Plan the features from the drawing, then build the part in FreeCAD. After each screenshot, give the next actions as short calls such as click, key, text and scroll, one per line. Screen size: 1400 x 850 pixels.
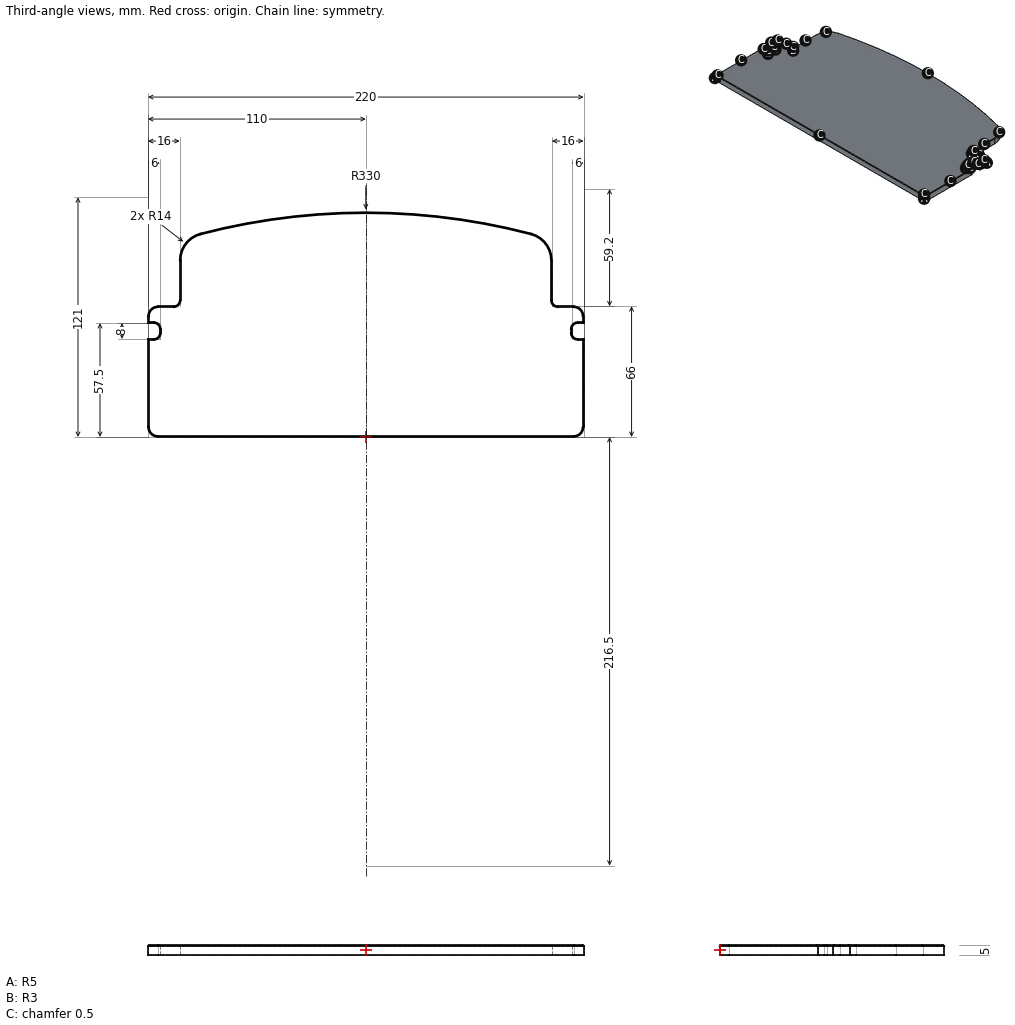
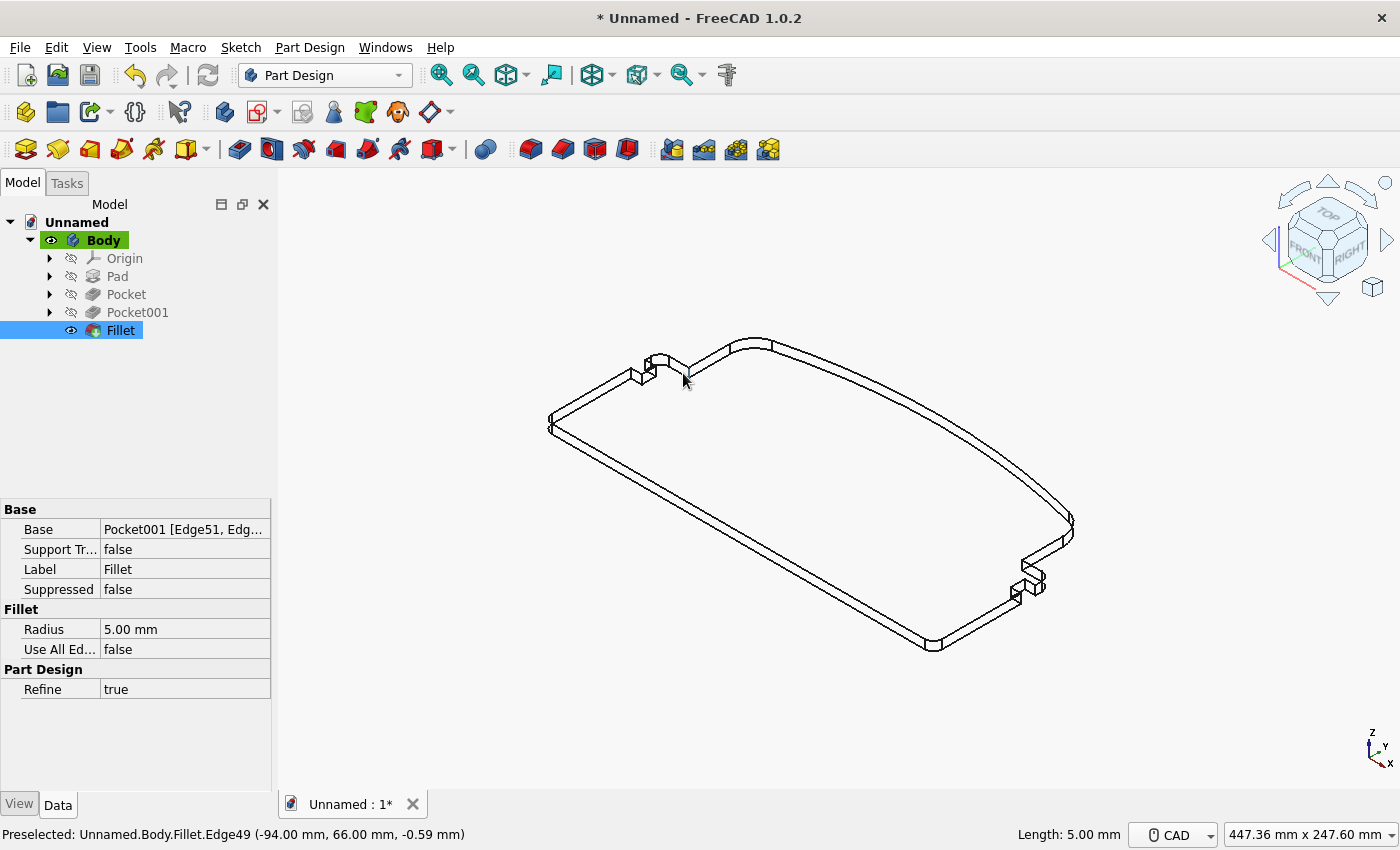
click(1022, 567, ctrl)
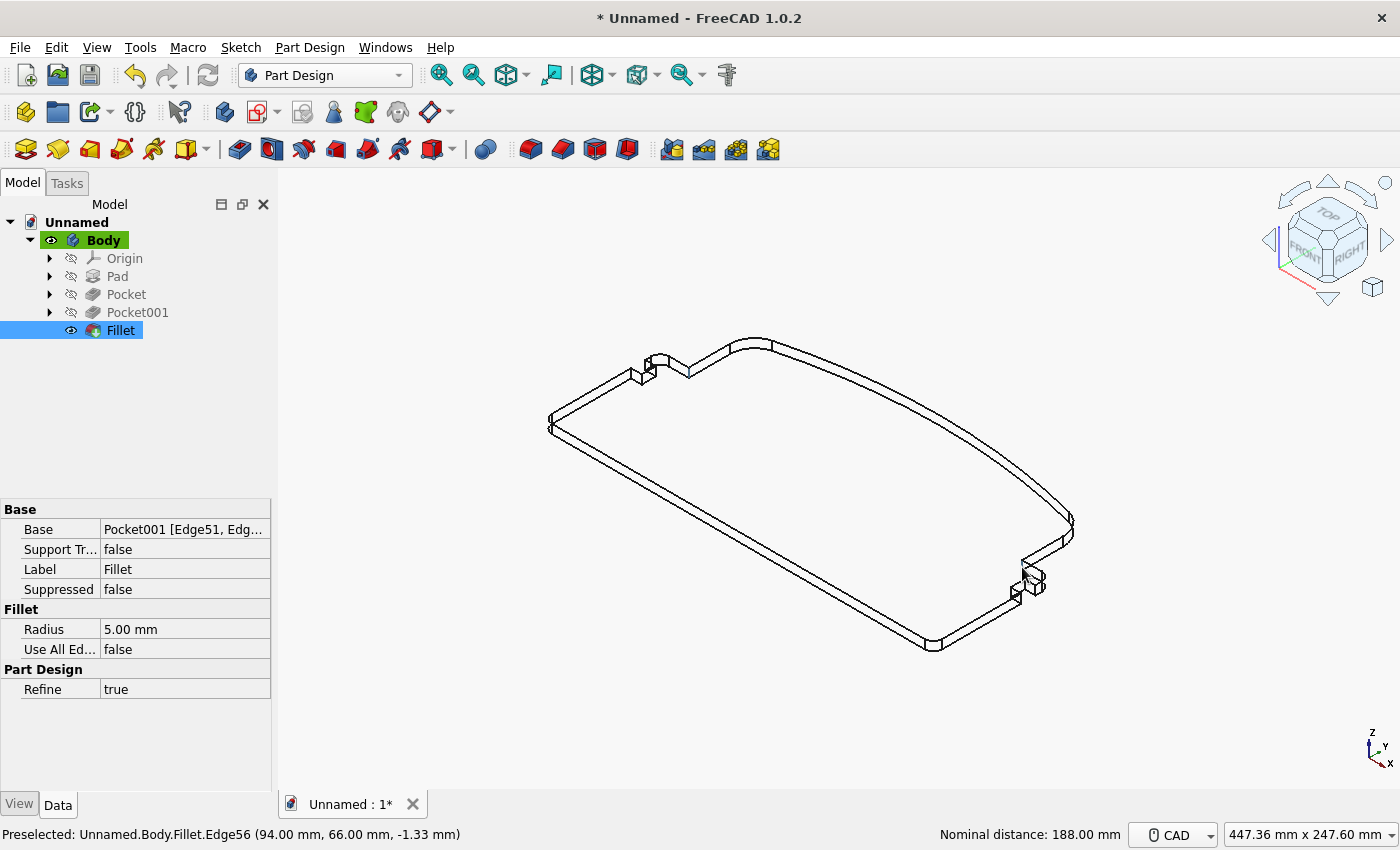
click(656, 373, ctrl)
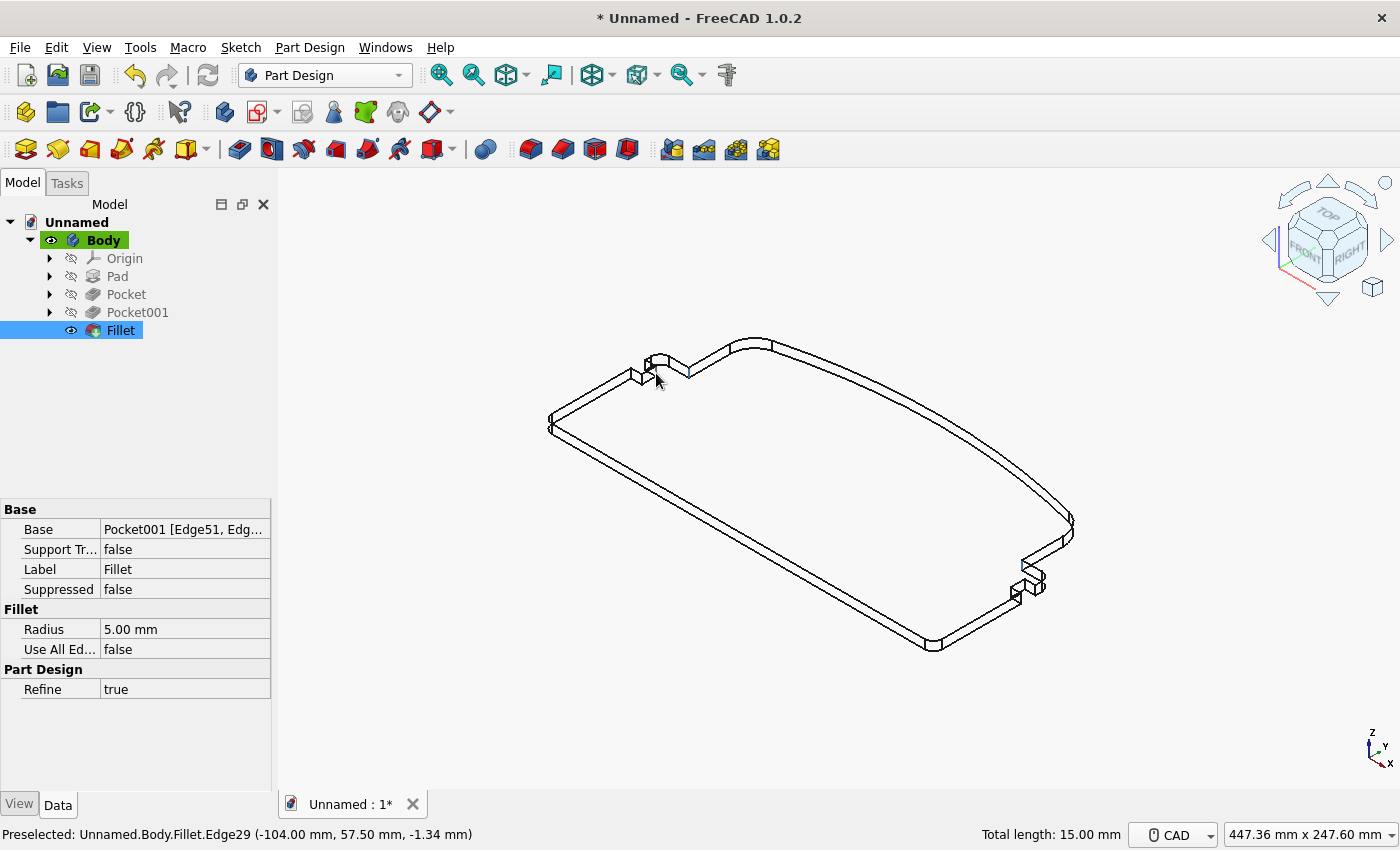
click(642, 380, ctrl)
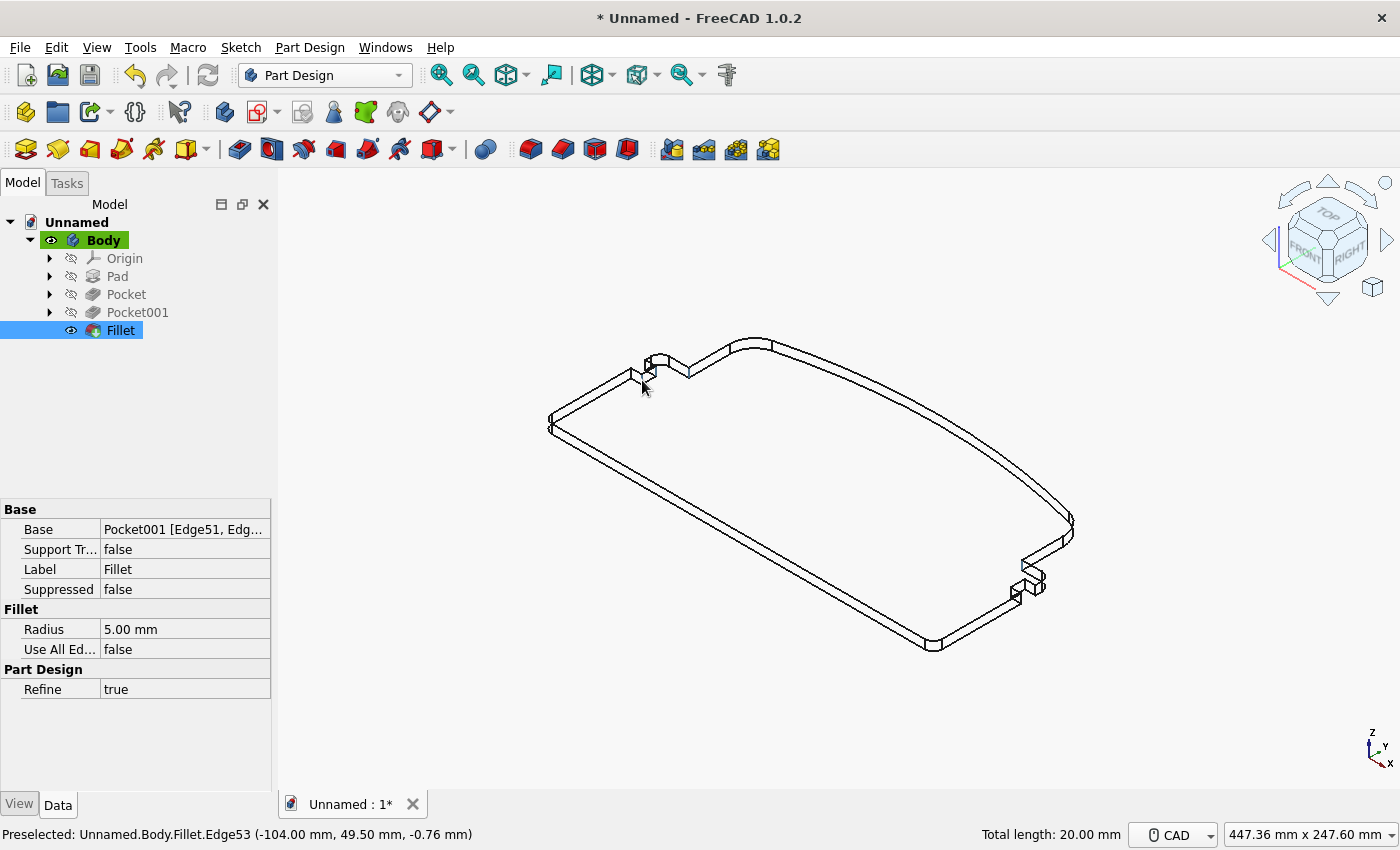
click(1025, 586, ctrl)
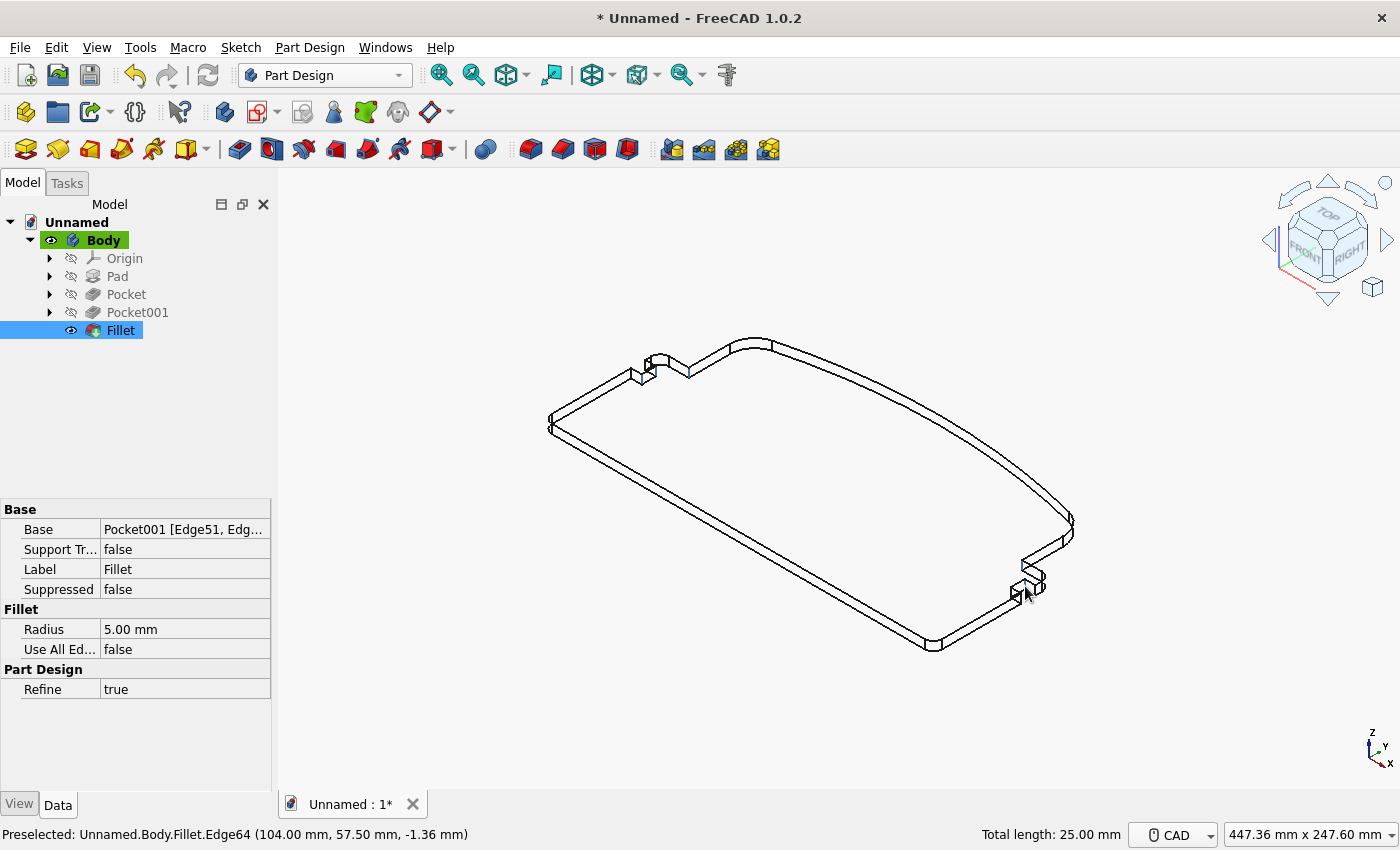
scroll(1011, 591, up, 6)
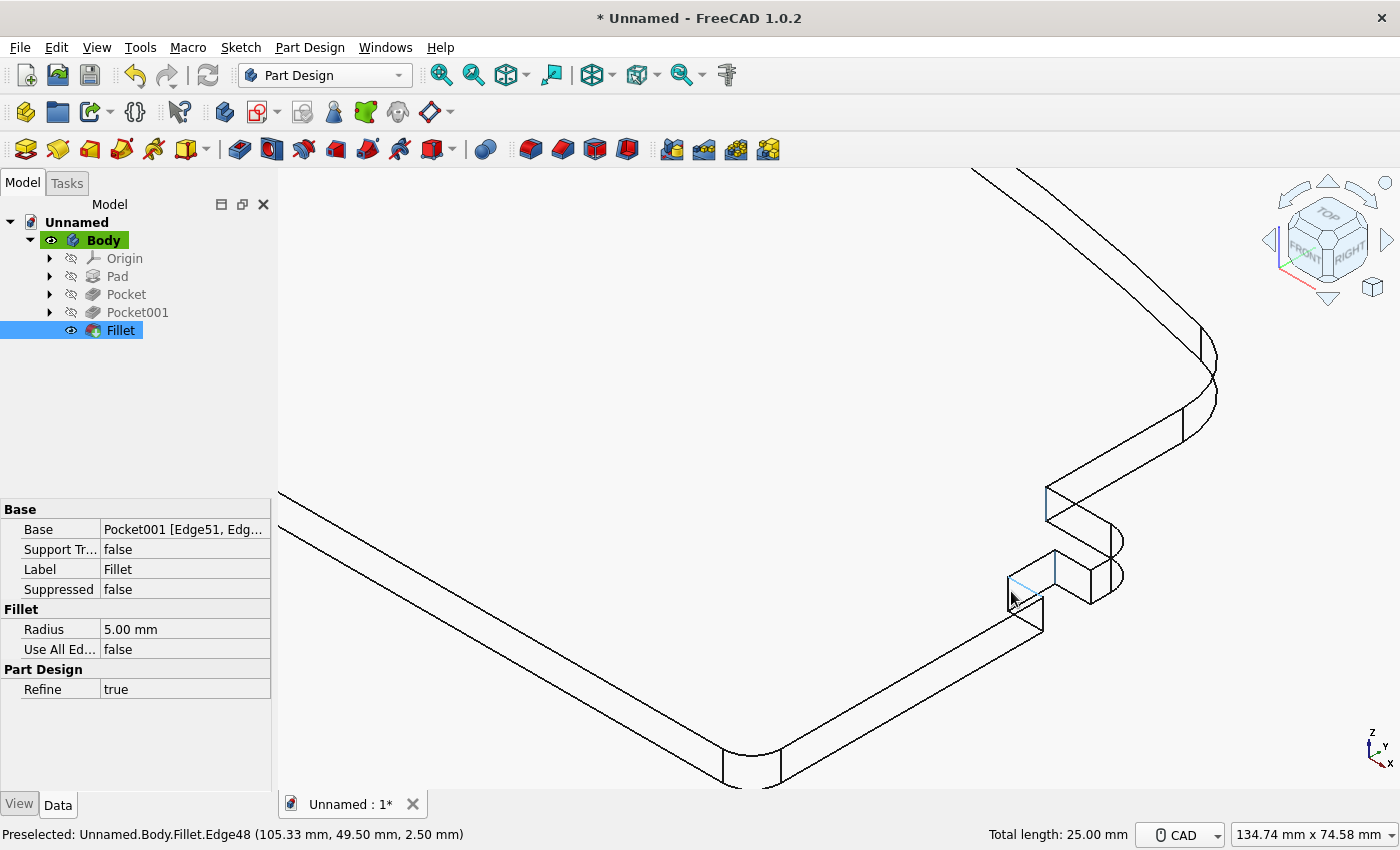
click(1008, 593, ctrl)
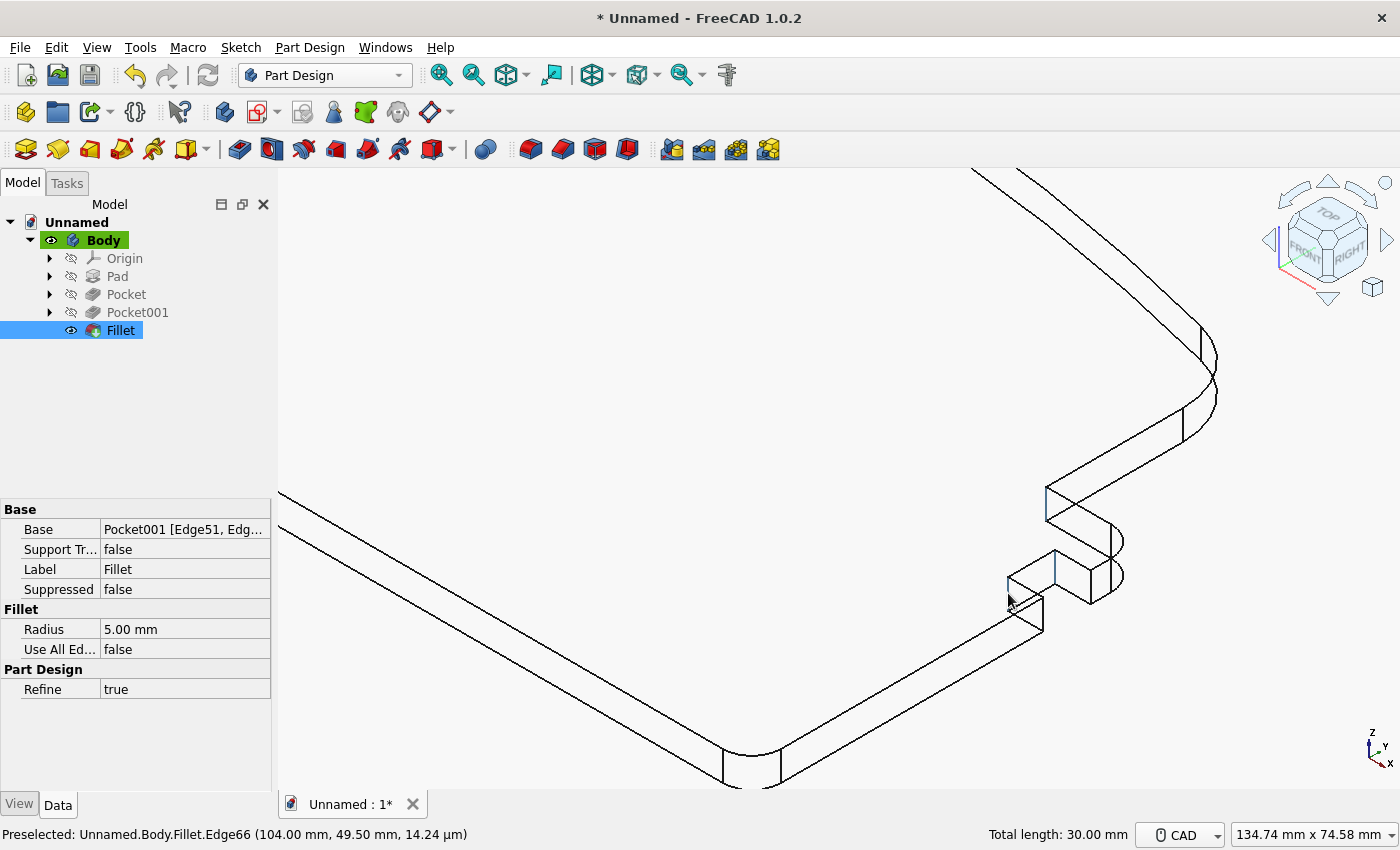
key(v)
key(1)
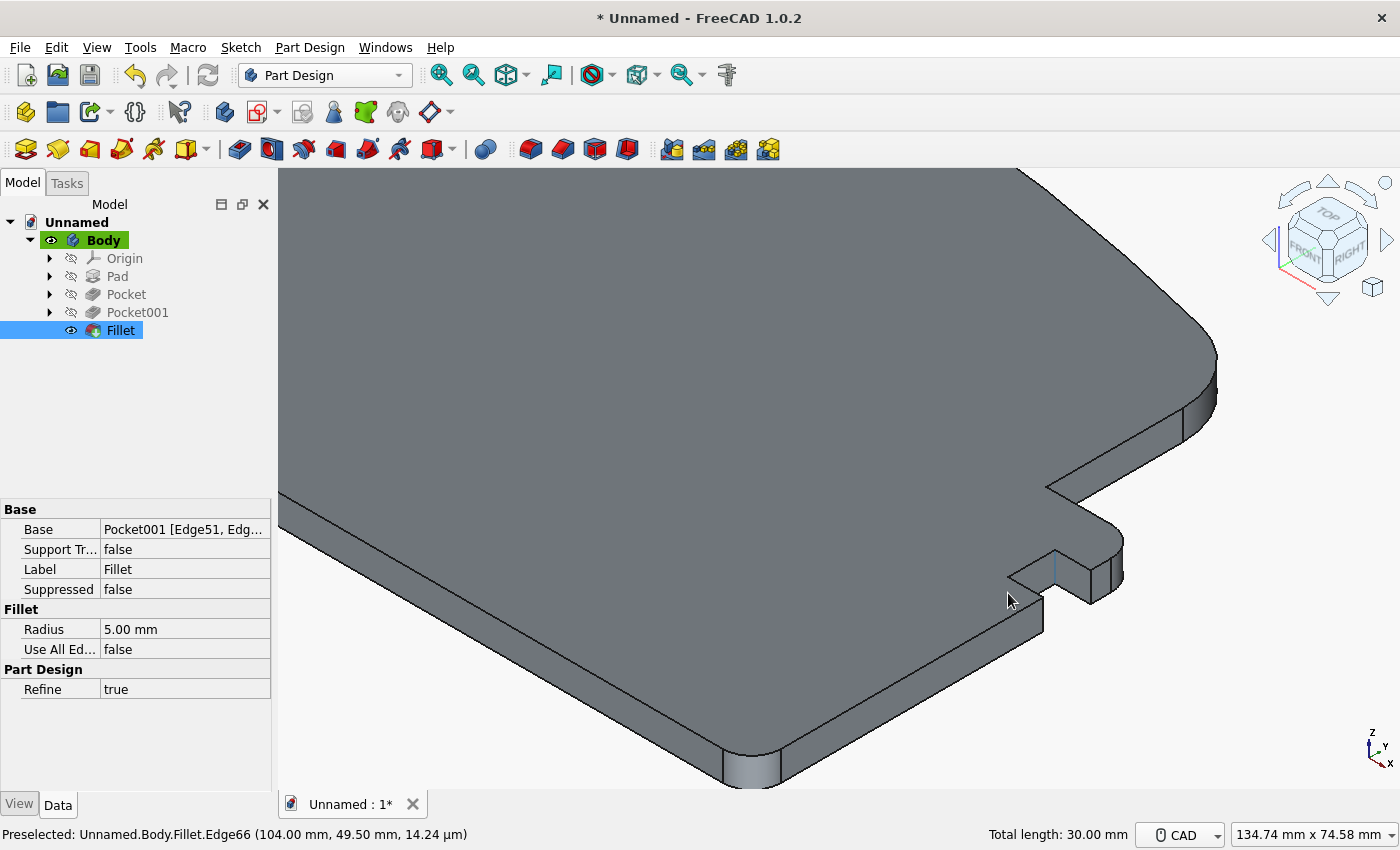
click(532, 150)